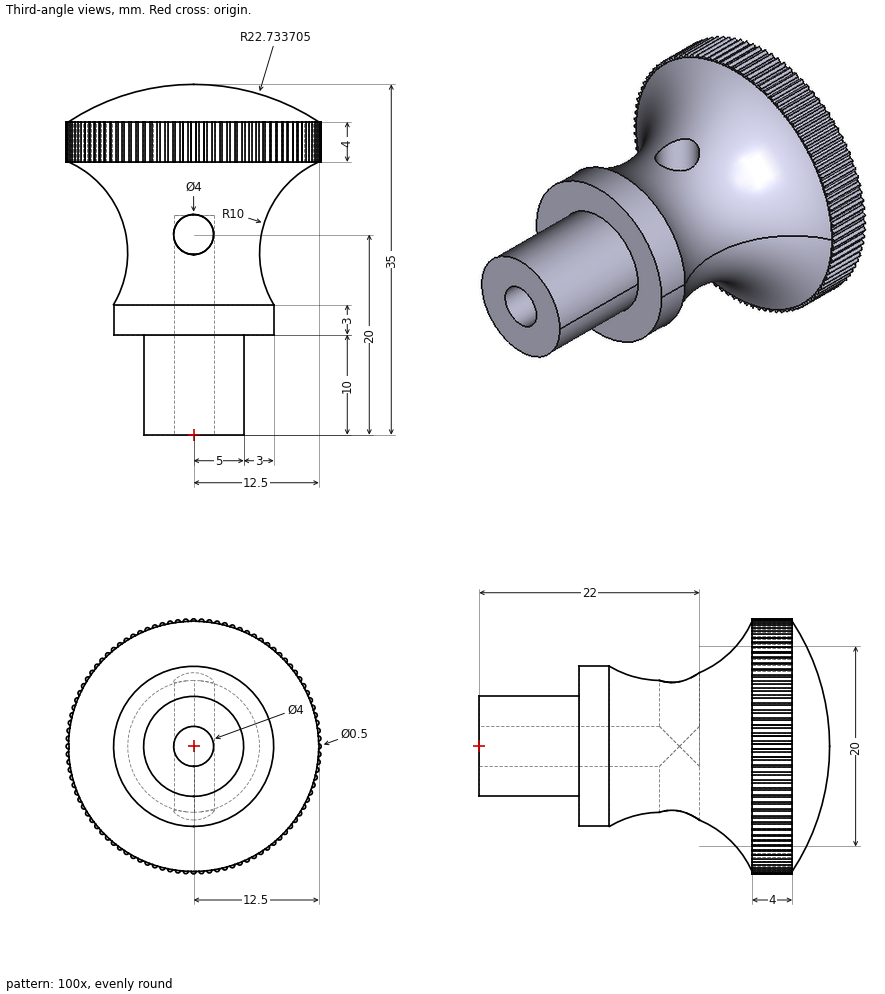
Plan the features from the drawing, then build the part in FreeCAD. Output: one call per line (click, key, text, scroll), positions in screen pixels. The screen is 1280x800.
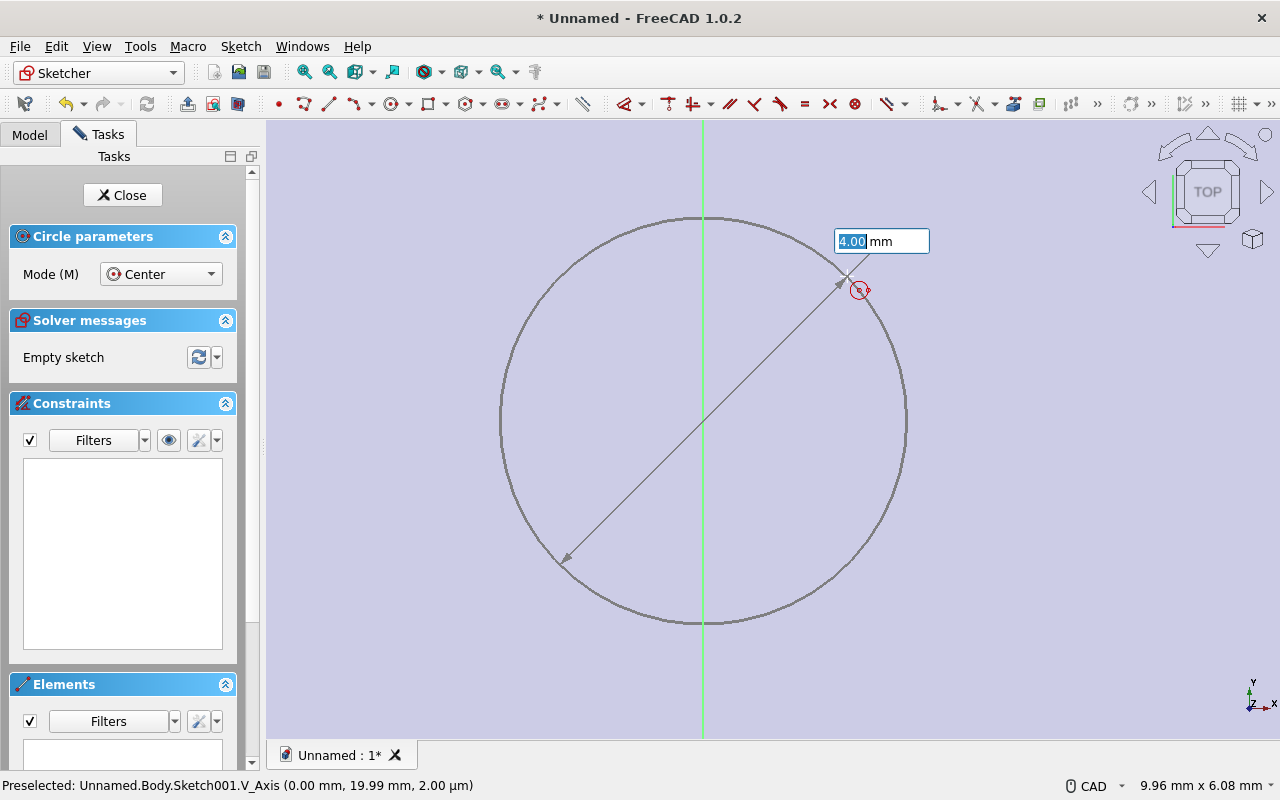
text(4)
key(Return)
key(Escape)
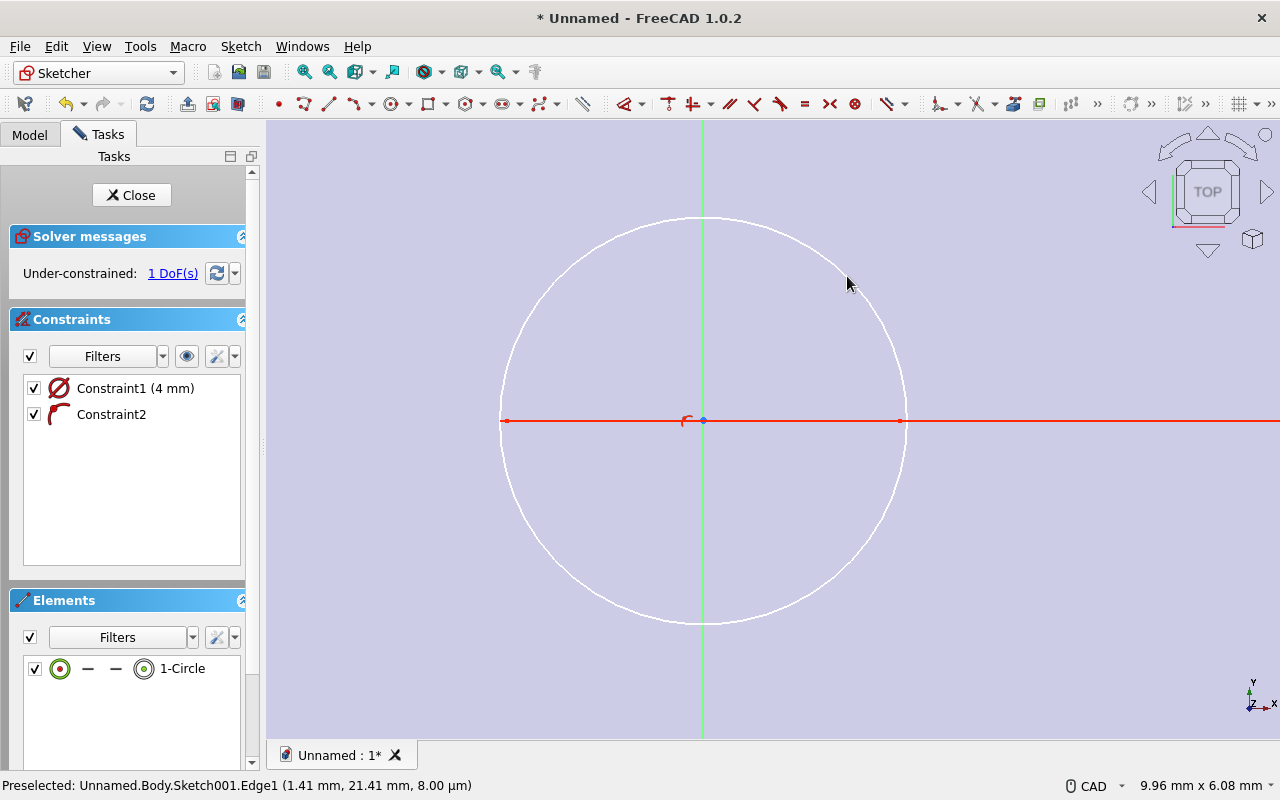
click(624, 104)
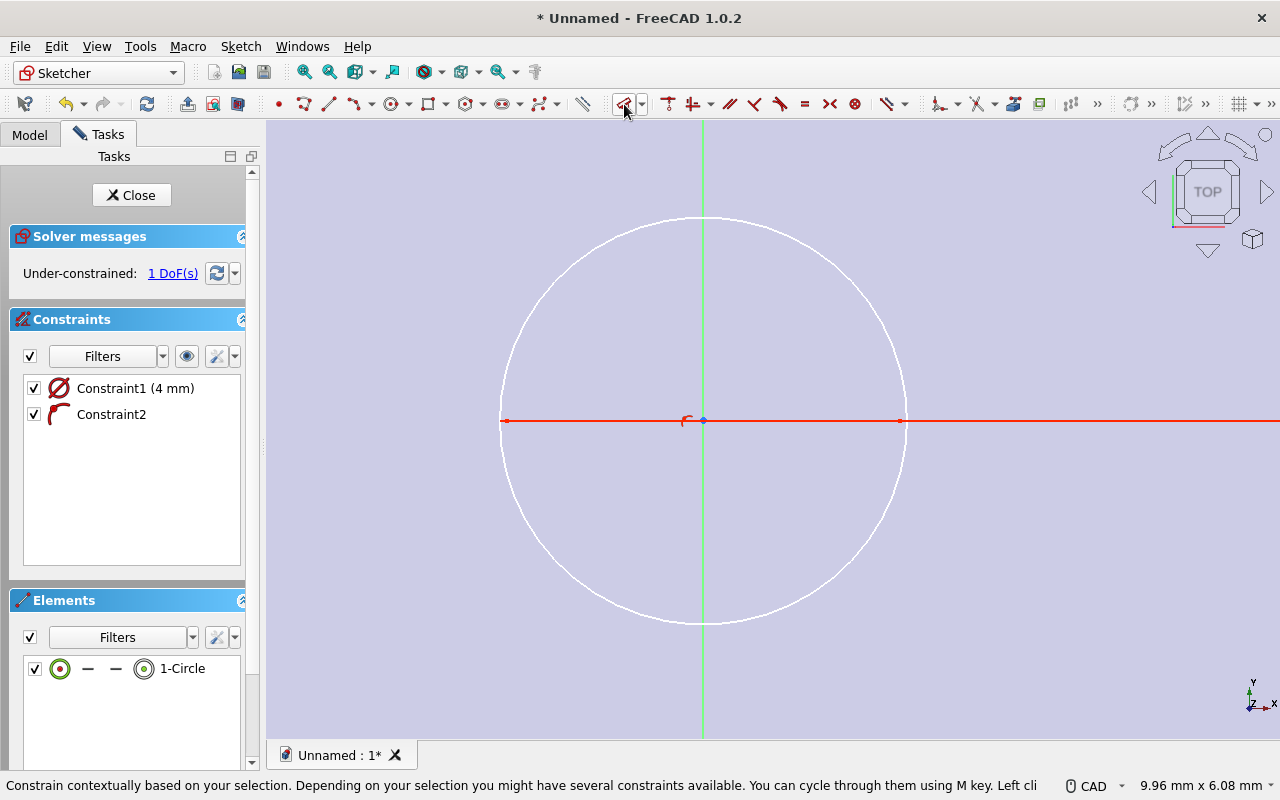
click(703, 421)
click(737, 566)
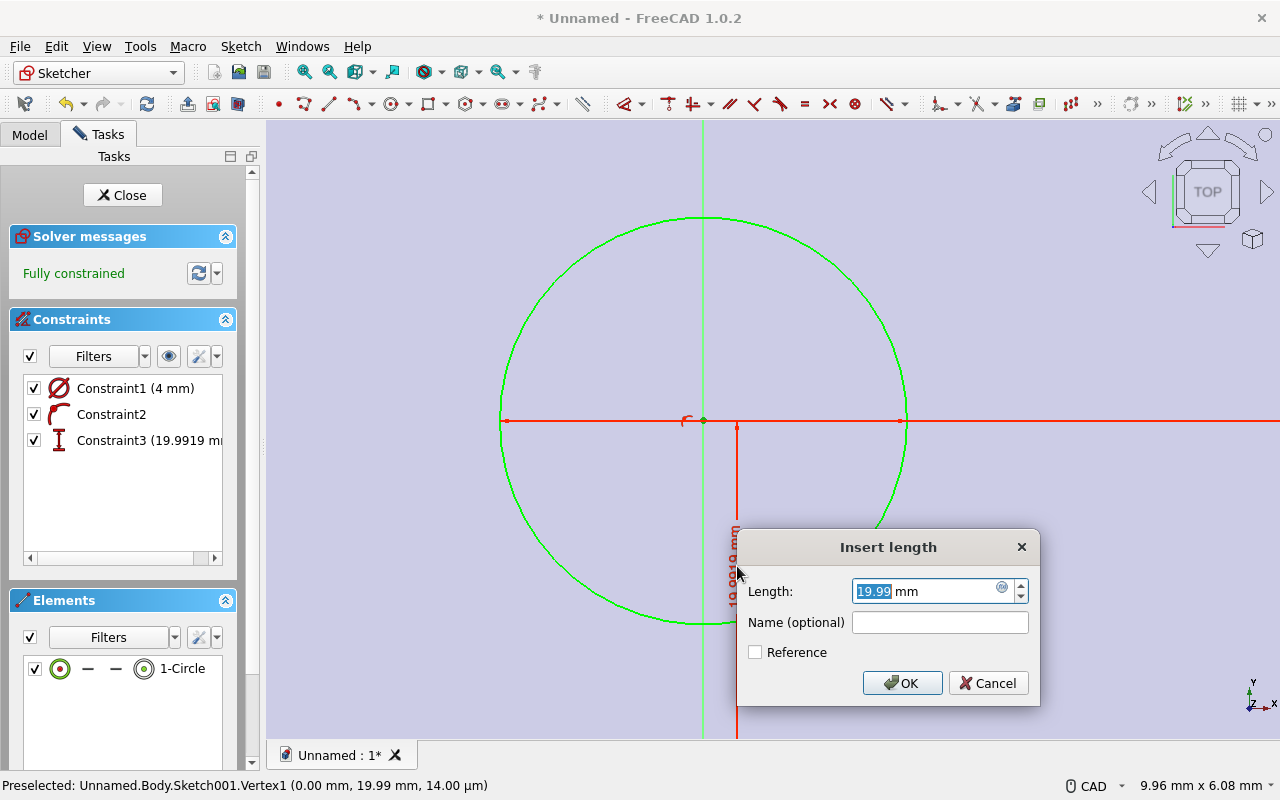
text(20)
key(Return)
key(Escape)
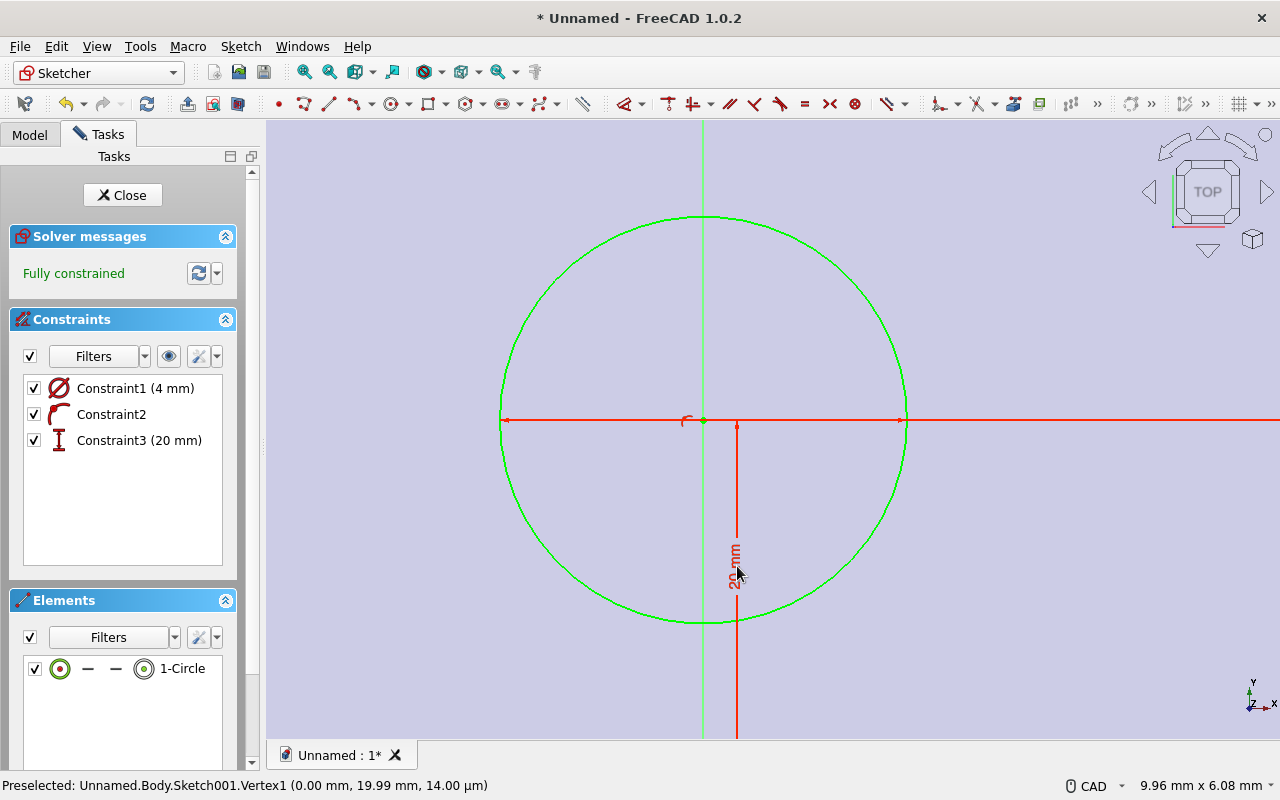
click(123, 195)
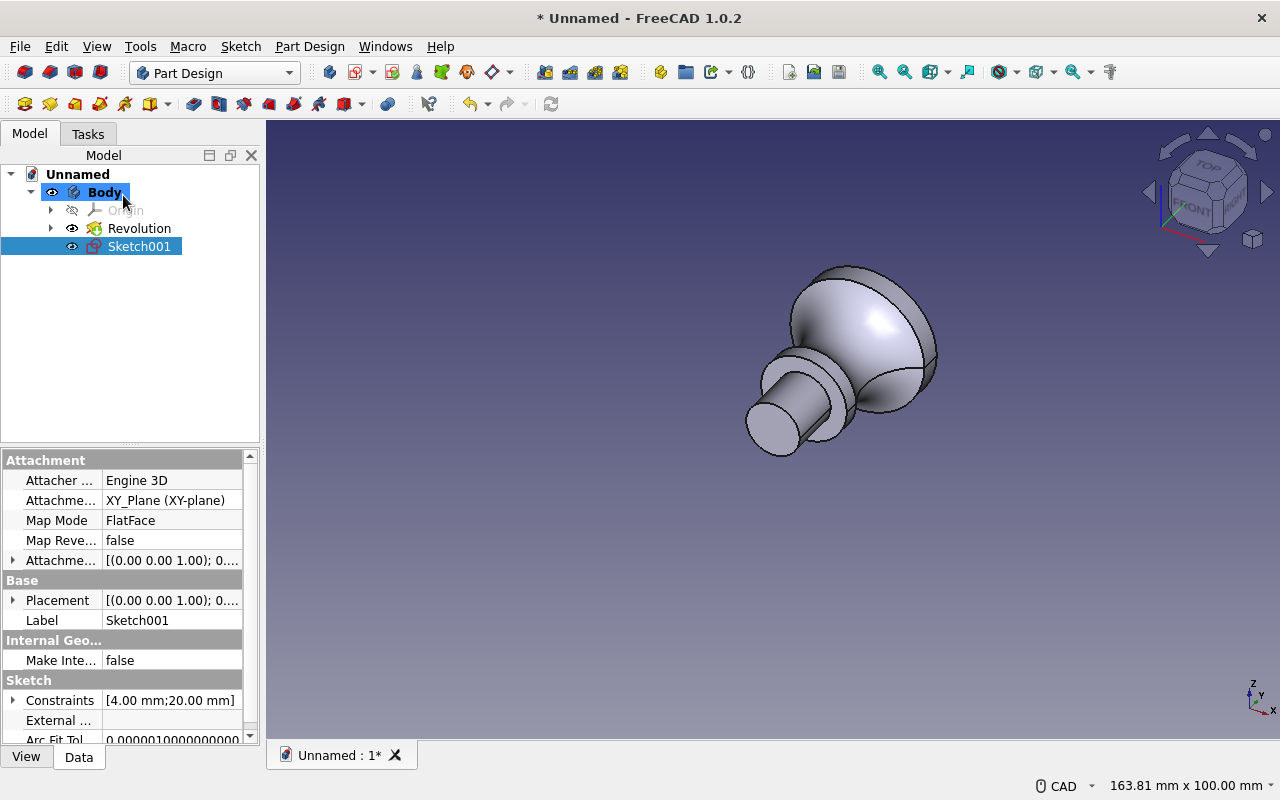
click(194, 104)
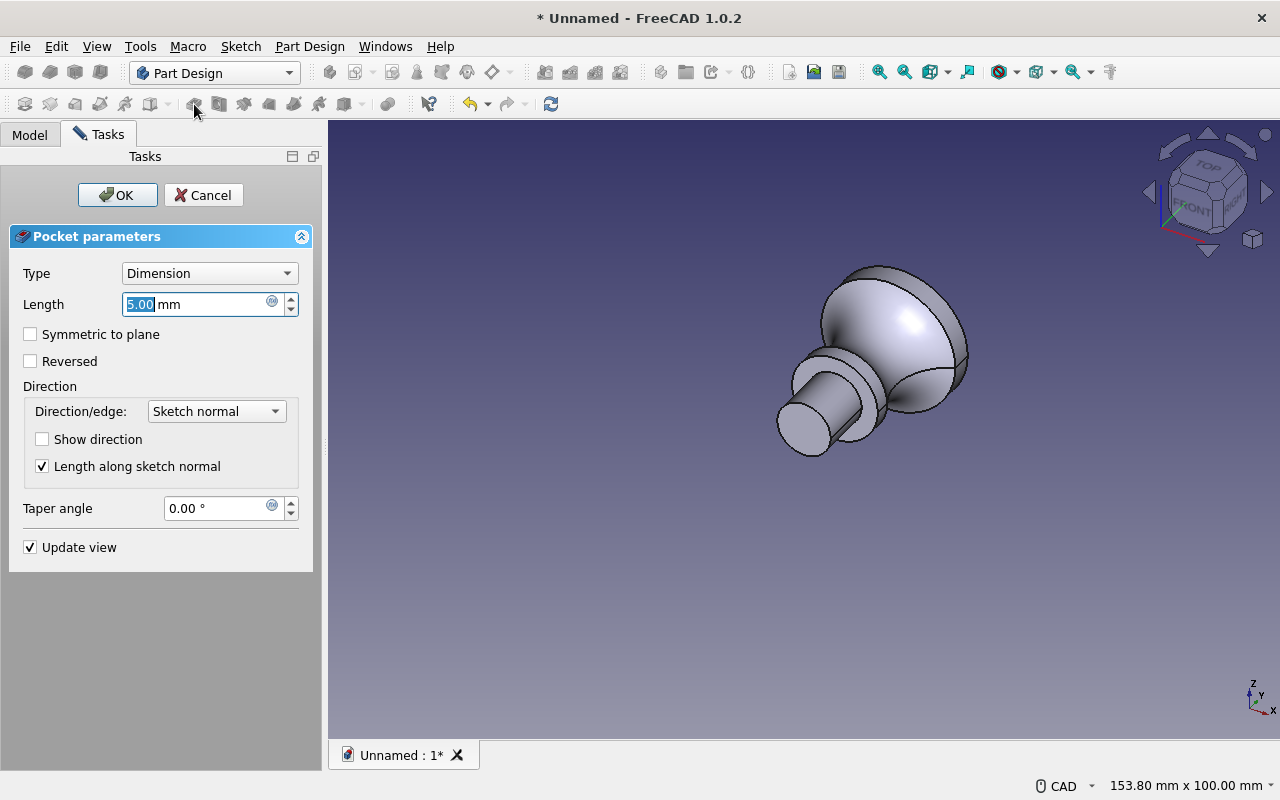
text(20)
key(Tab)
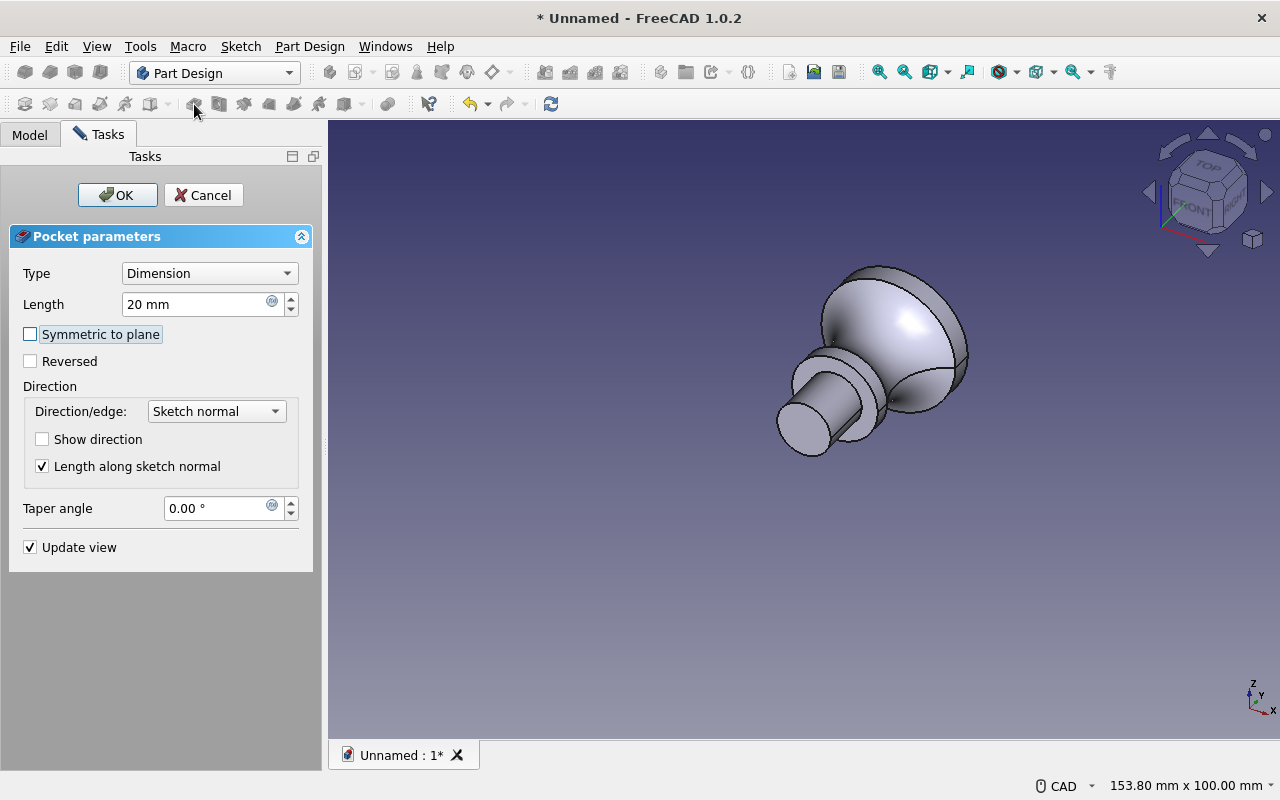
click(31, 334)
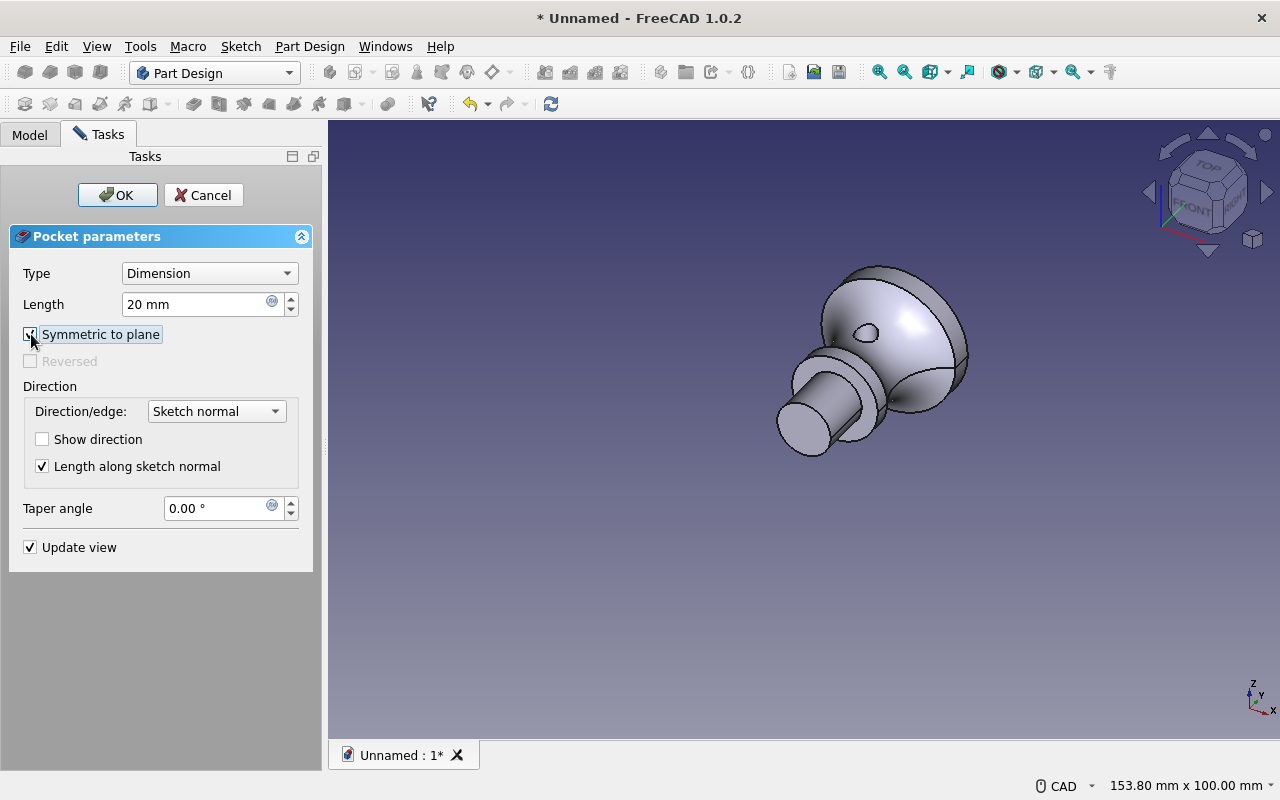
click(118, 195)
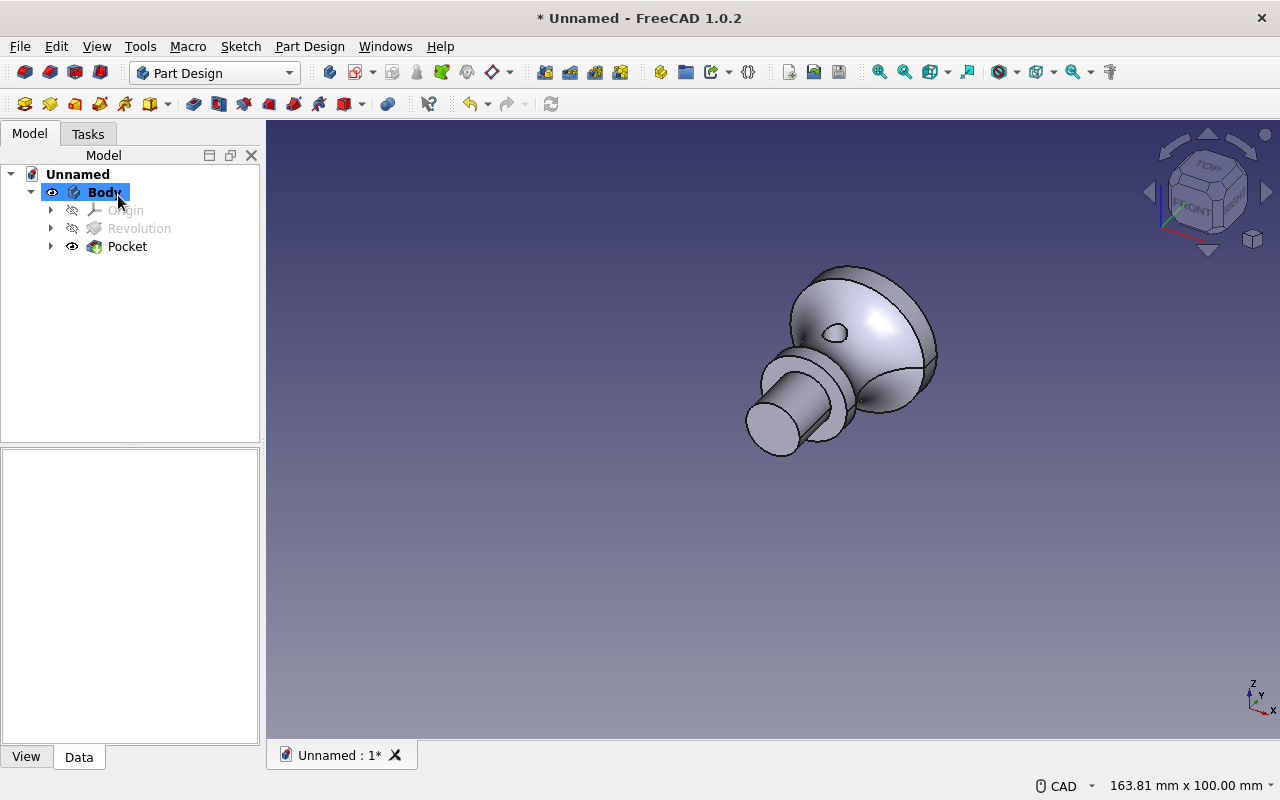
click(51, 210)